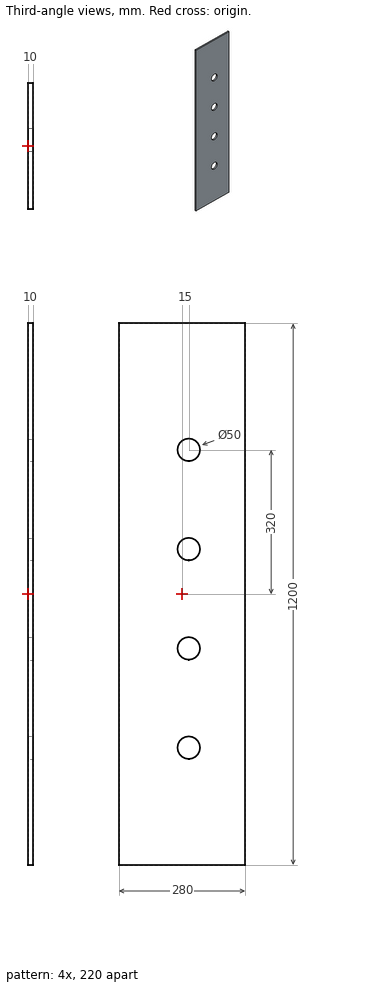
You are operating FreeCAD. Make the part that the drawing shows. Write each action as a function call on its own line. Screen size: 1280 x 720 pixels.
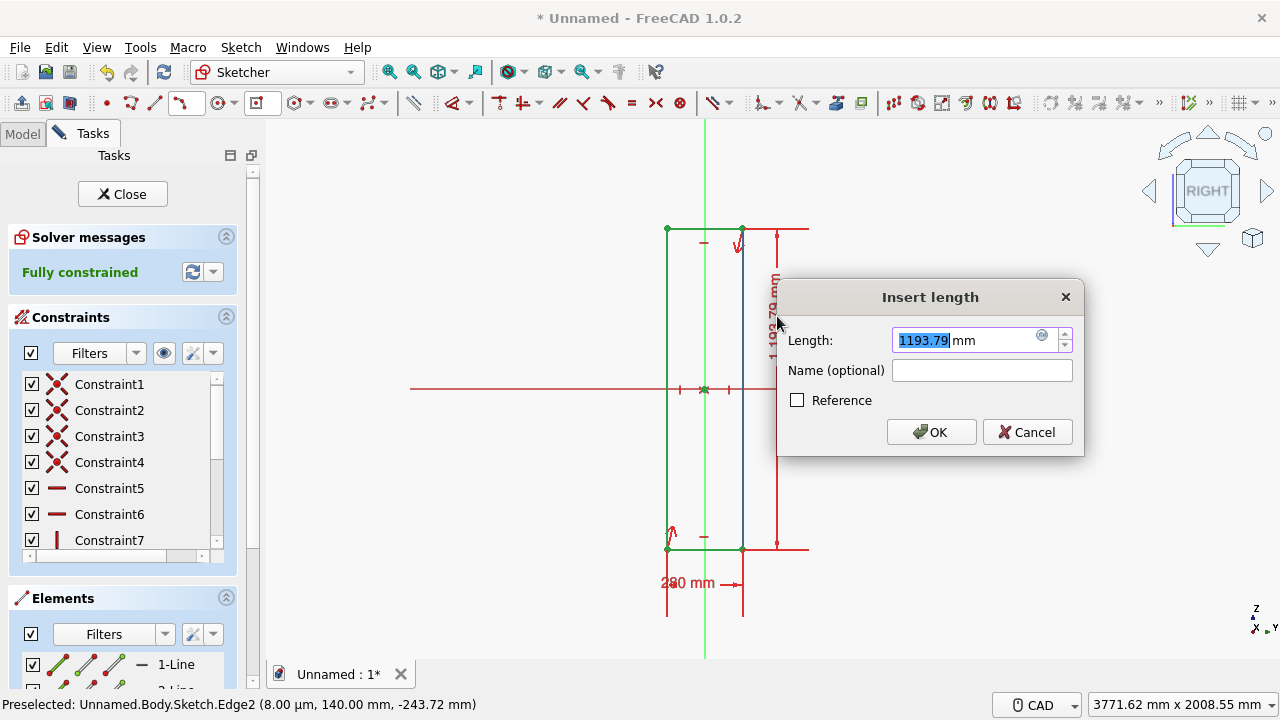
text(1200)
key(Return)
key(Escape)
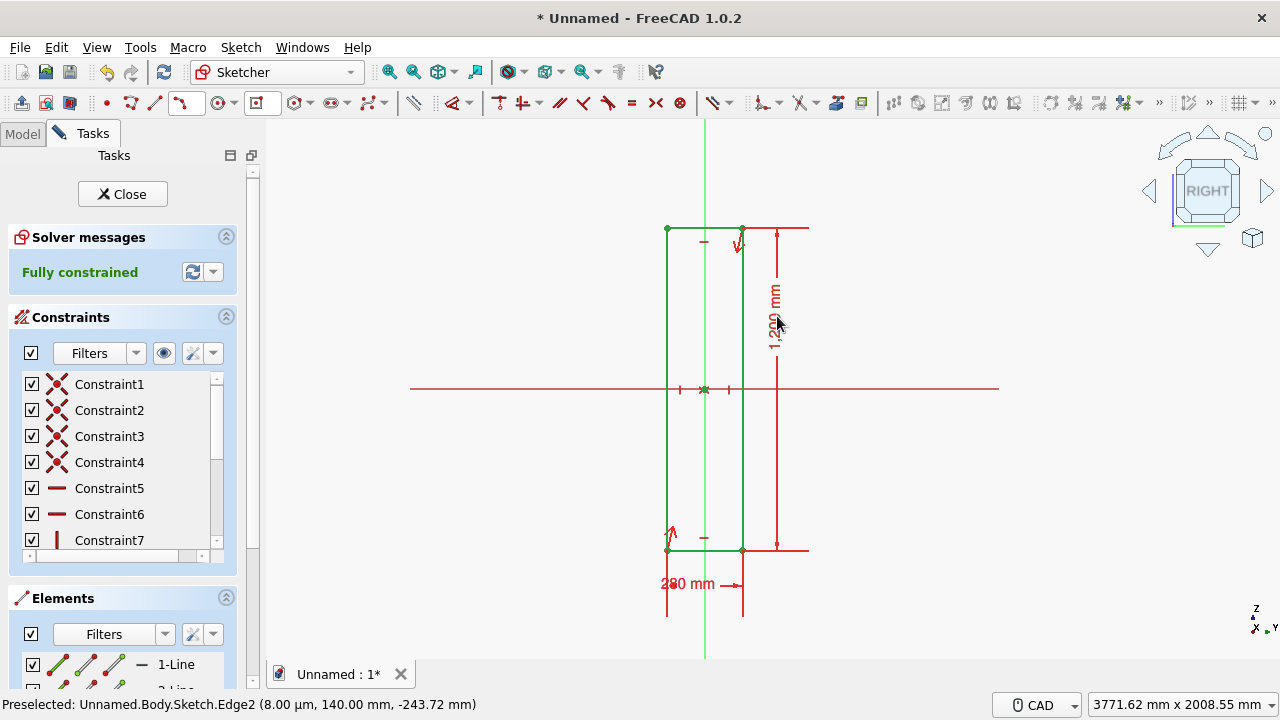
click(123, 194)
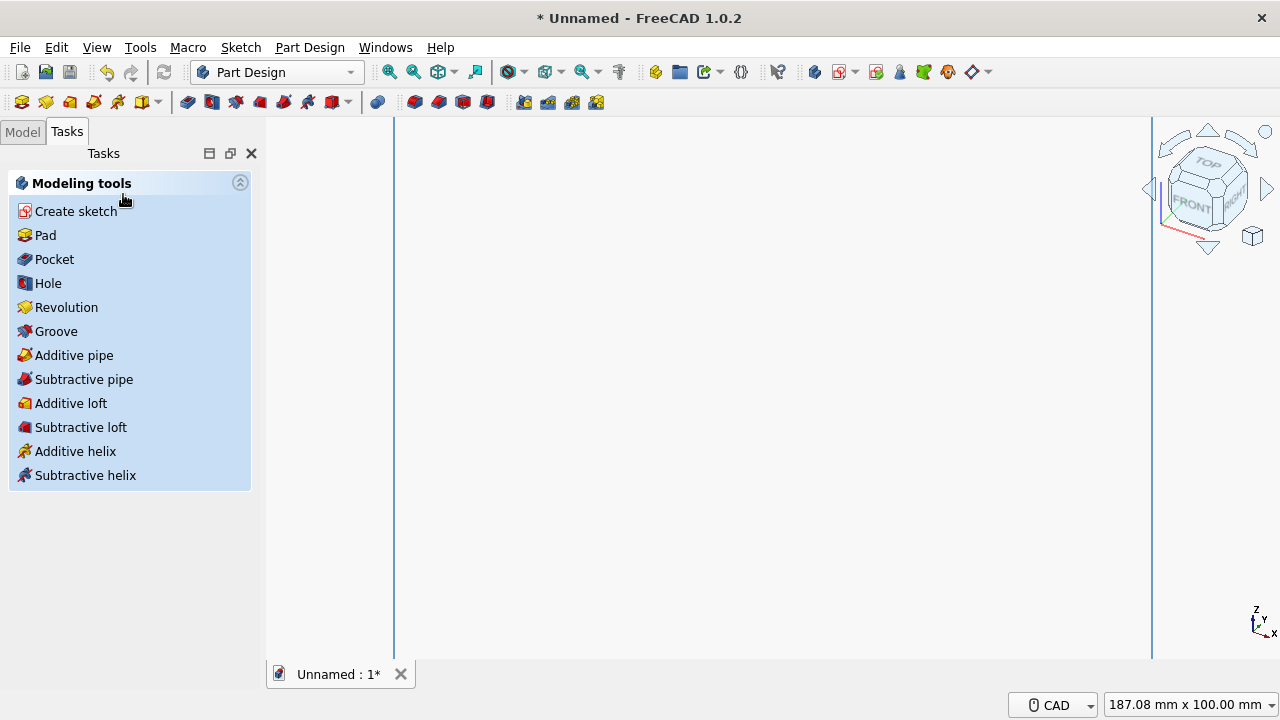
click(22, 102)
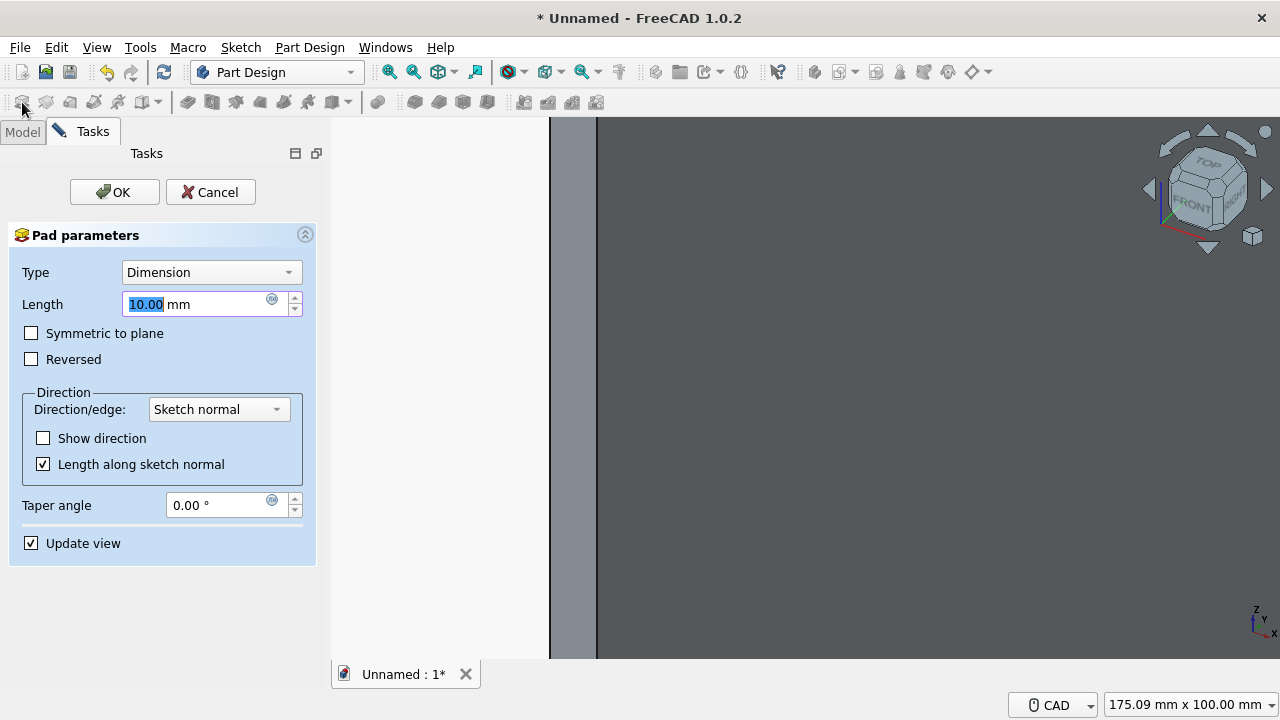
text(10)
key(Tab)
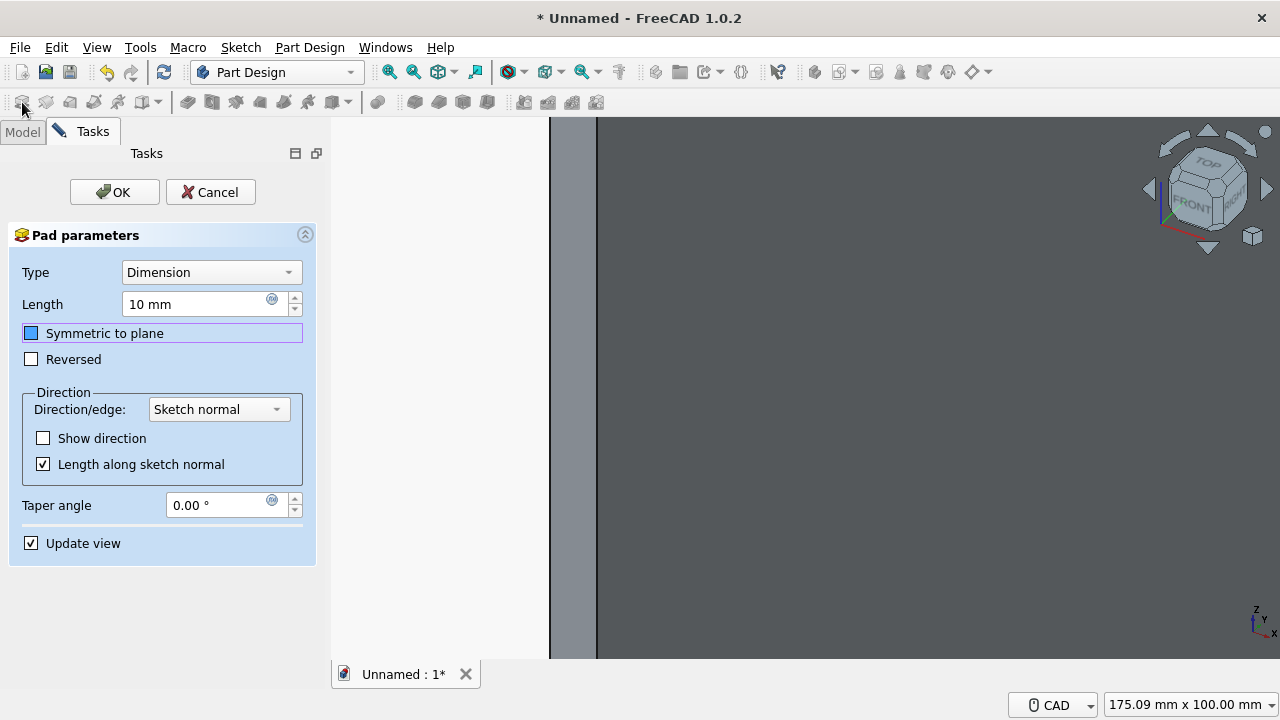
click(115, 192)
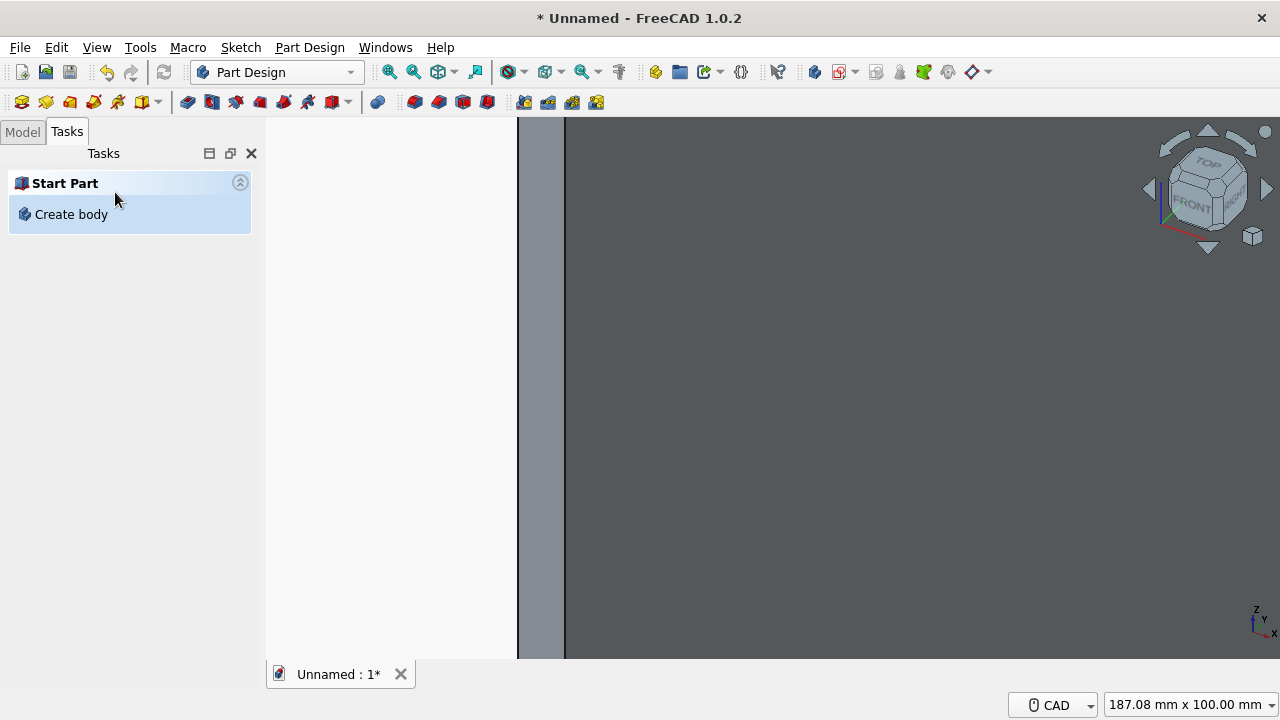
click(390, 72)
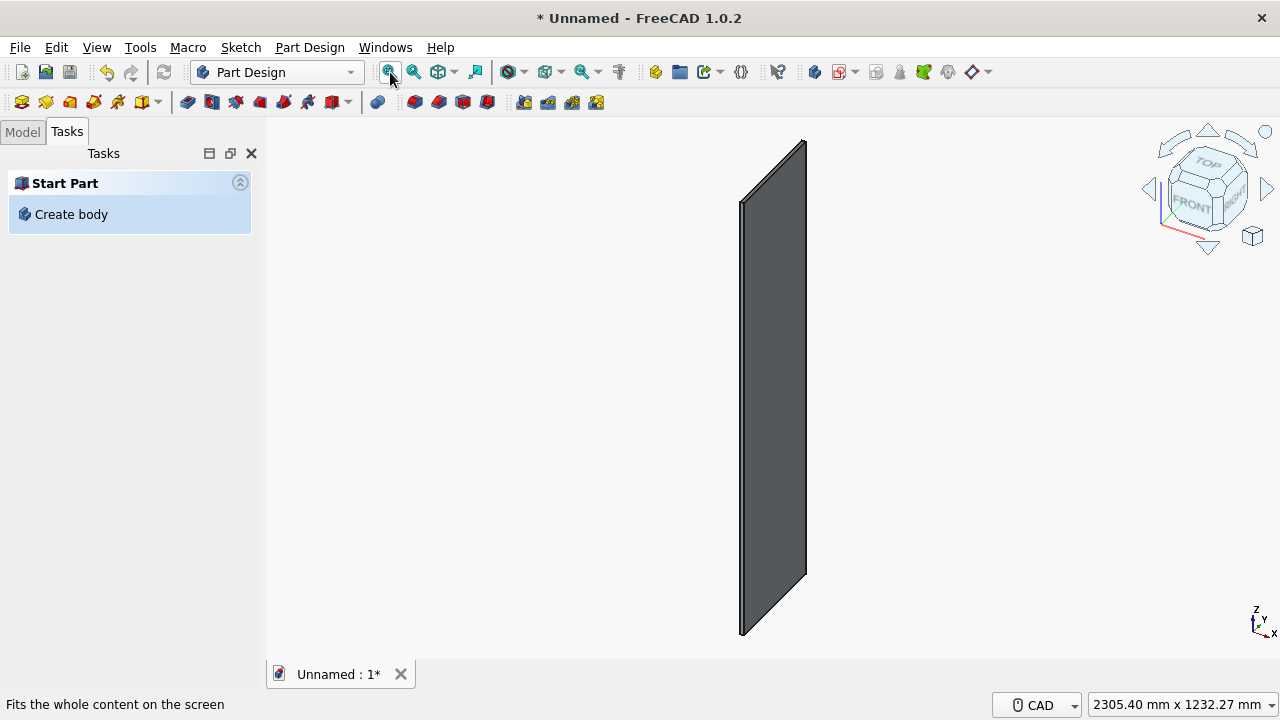
click(775, 511)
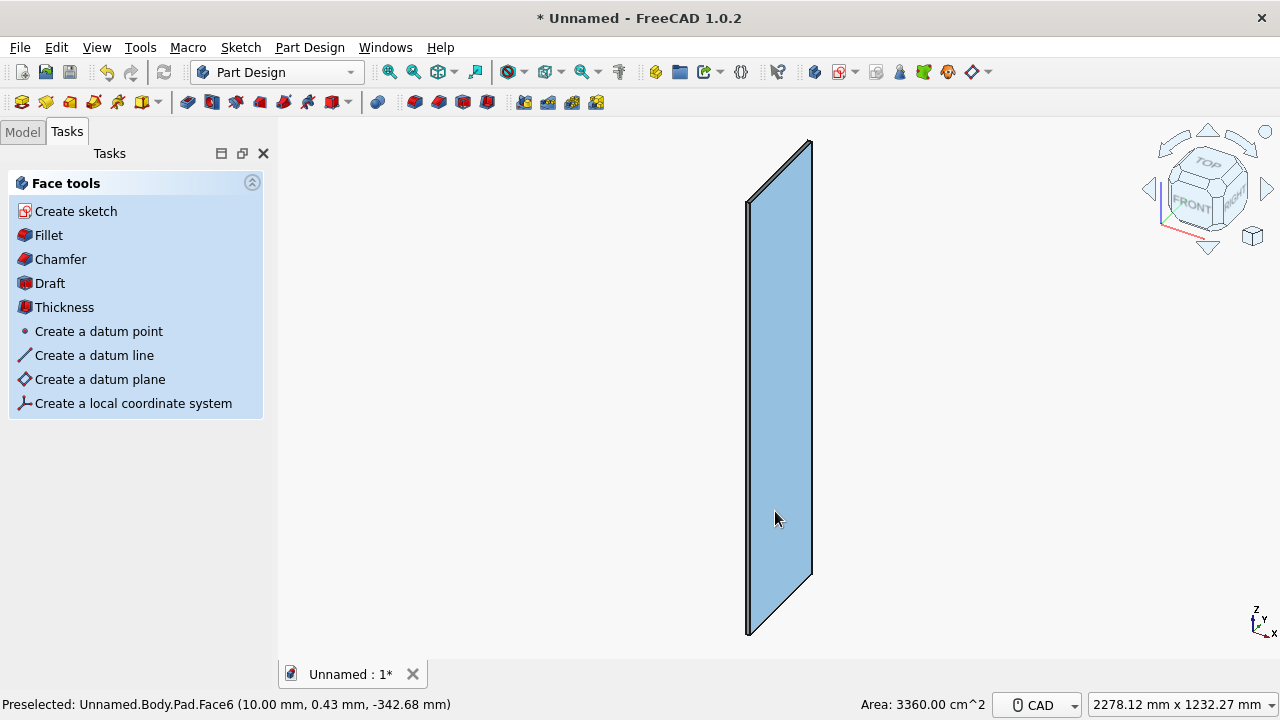
click(840, 72)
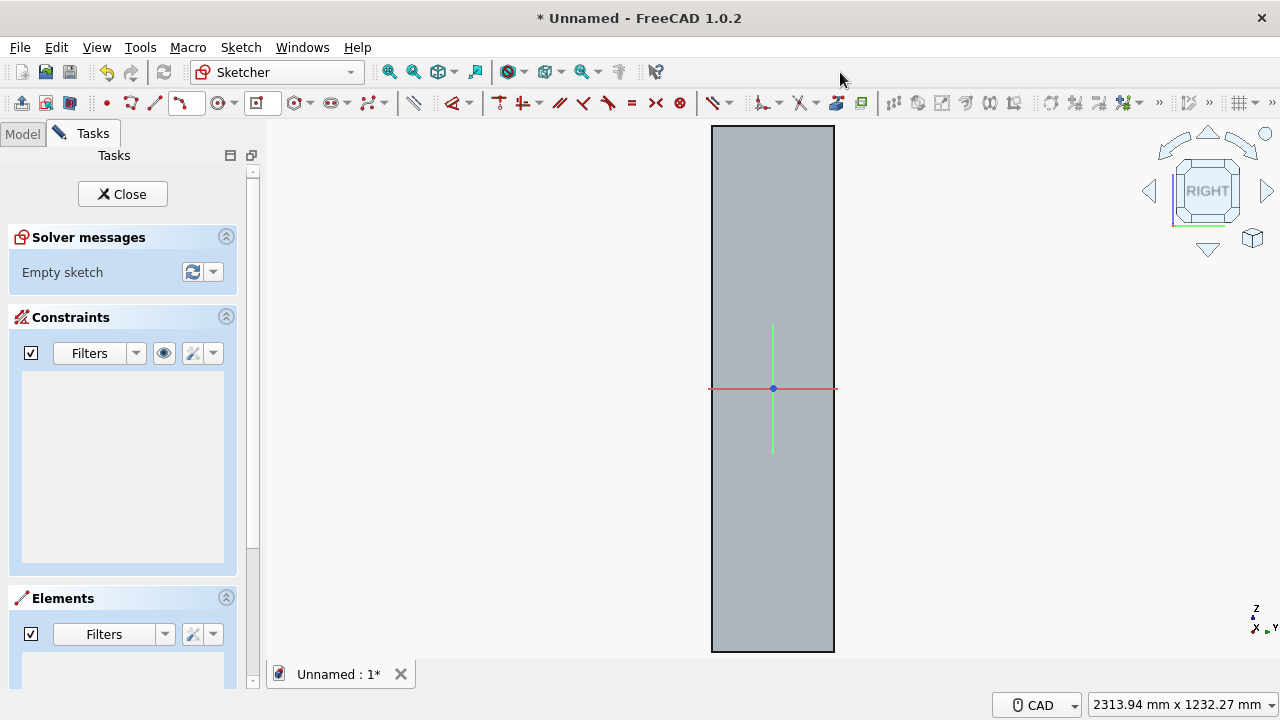
scroll(784, 240, up, 14)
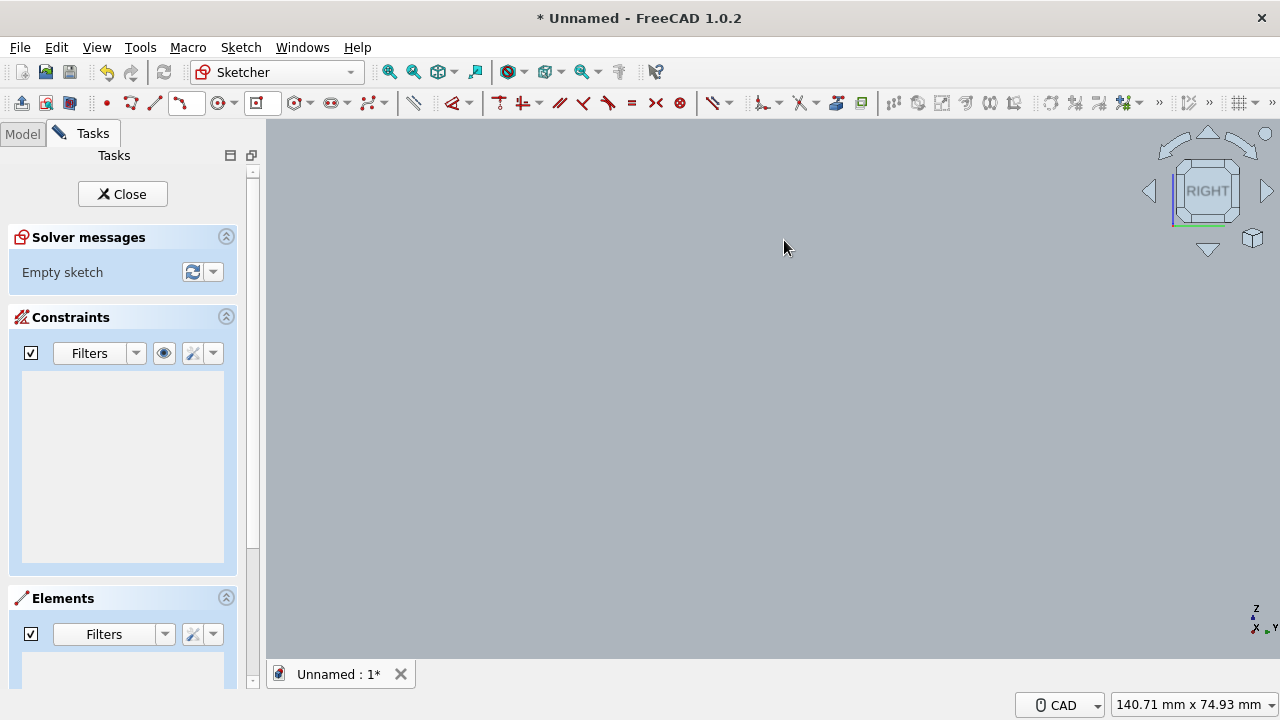
click(218, 104)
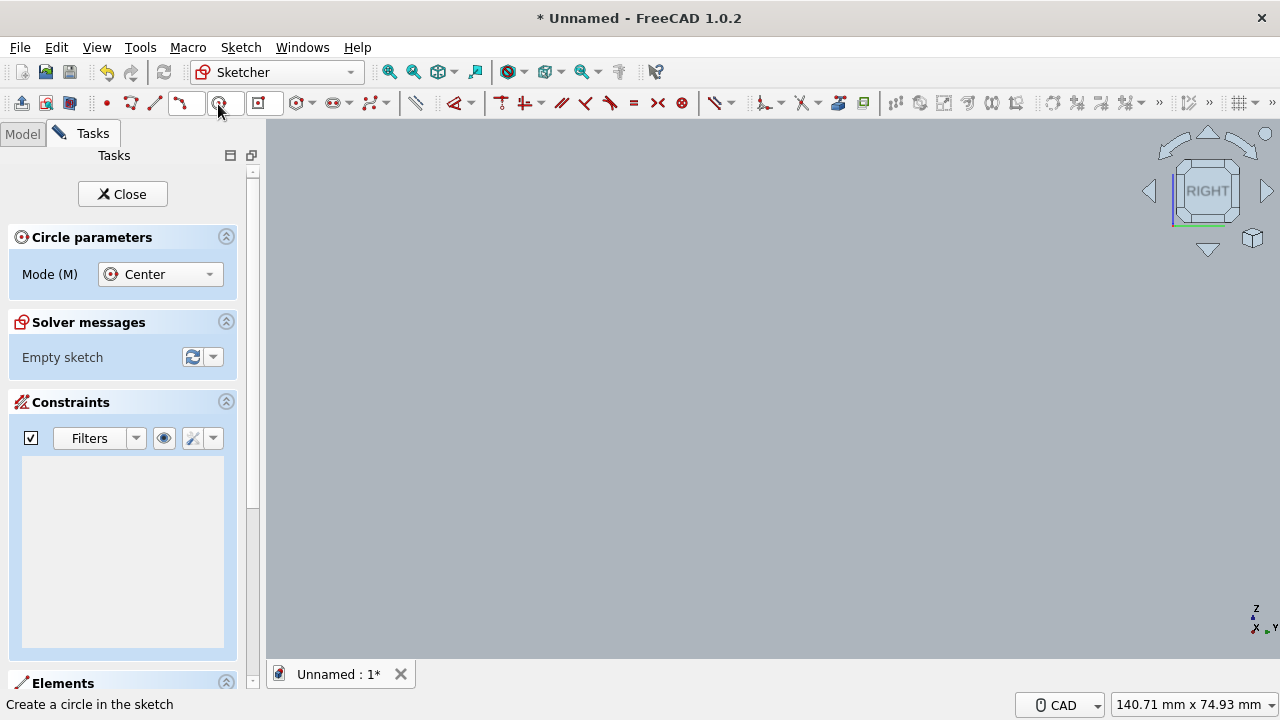
click(703, 381)
click(831, 253)
key(Escape)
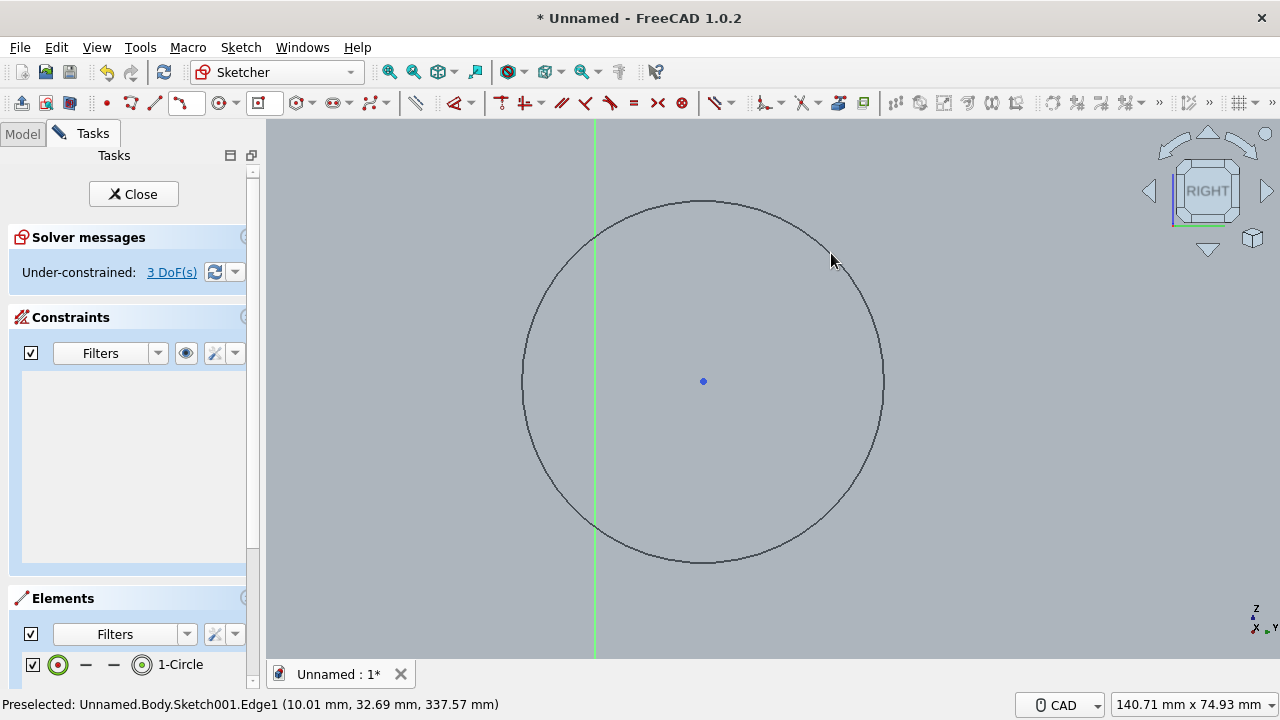
click(454, 104)